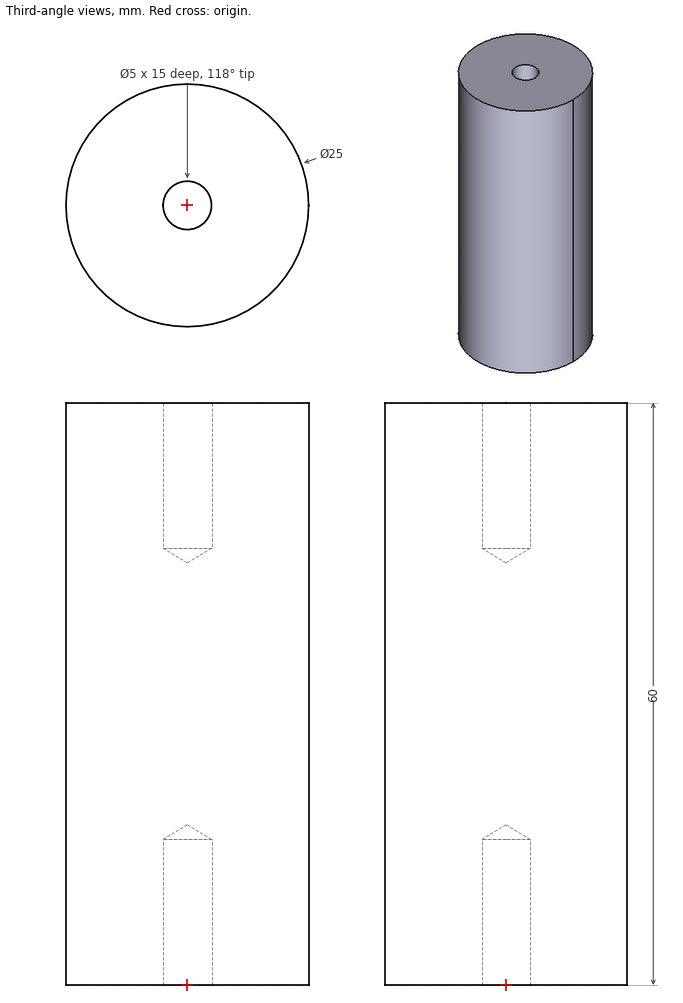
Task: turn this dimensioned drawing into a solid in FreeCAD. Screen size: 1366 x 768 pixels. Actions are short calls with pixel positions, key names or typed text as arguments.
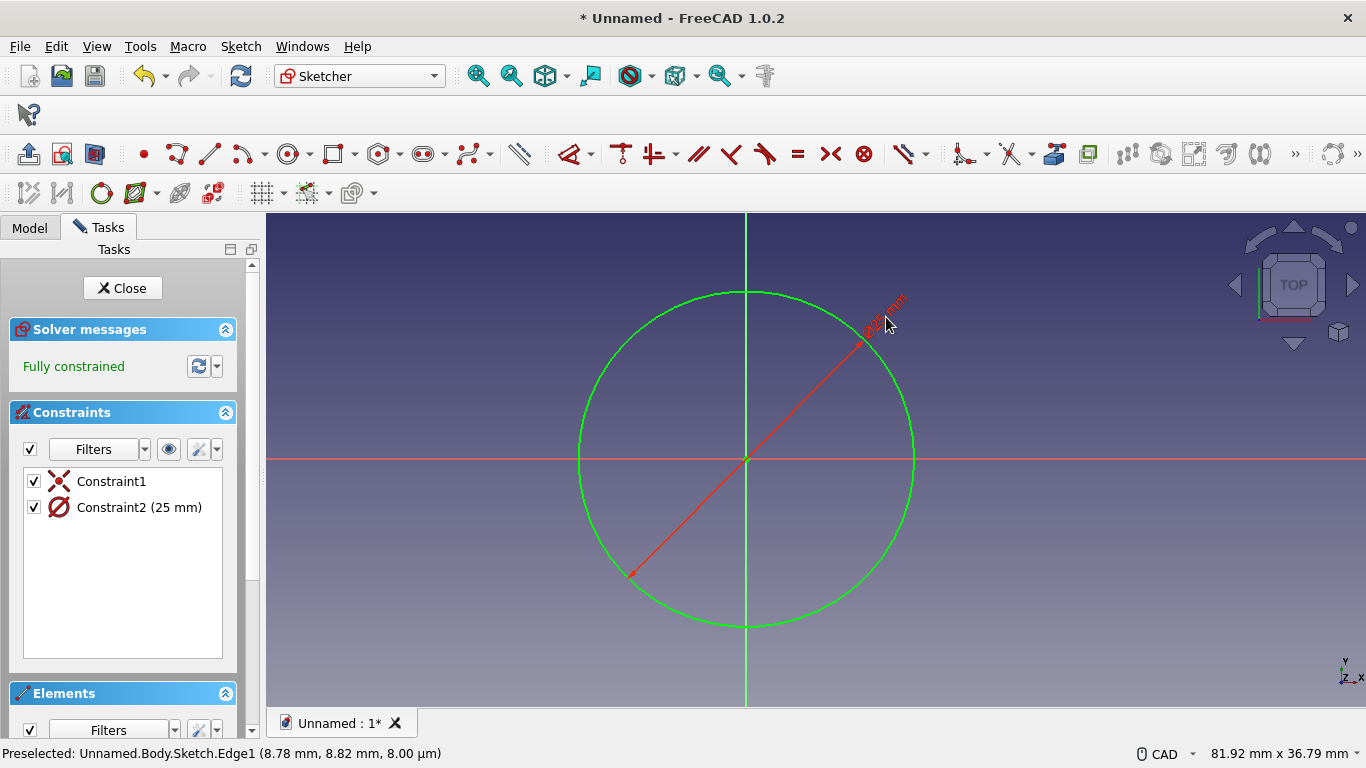
click(123, 288)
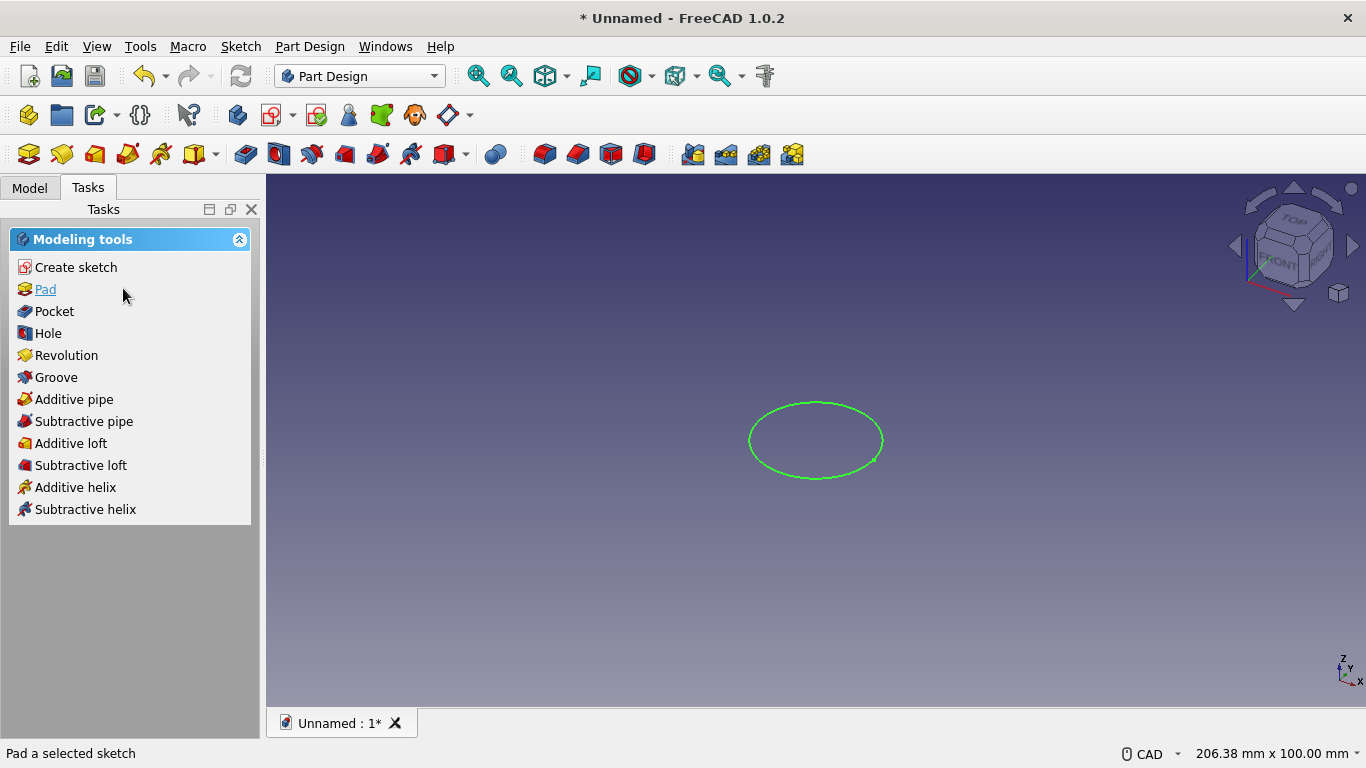
click(29, 154)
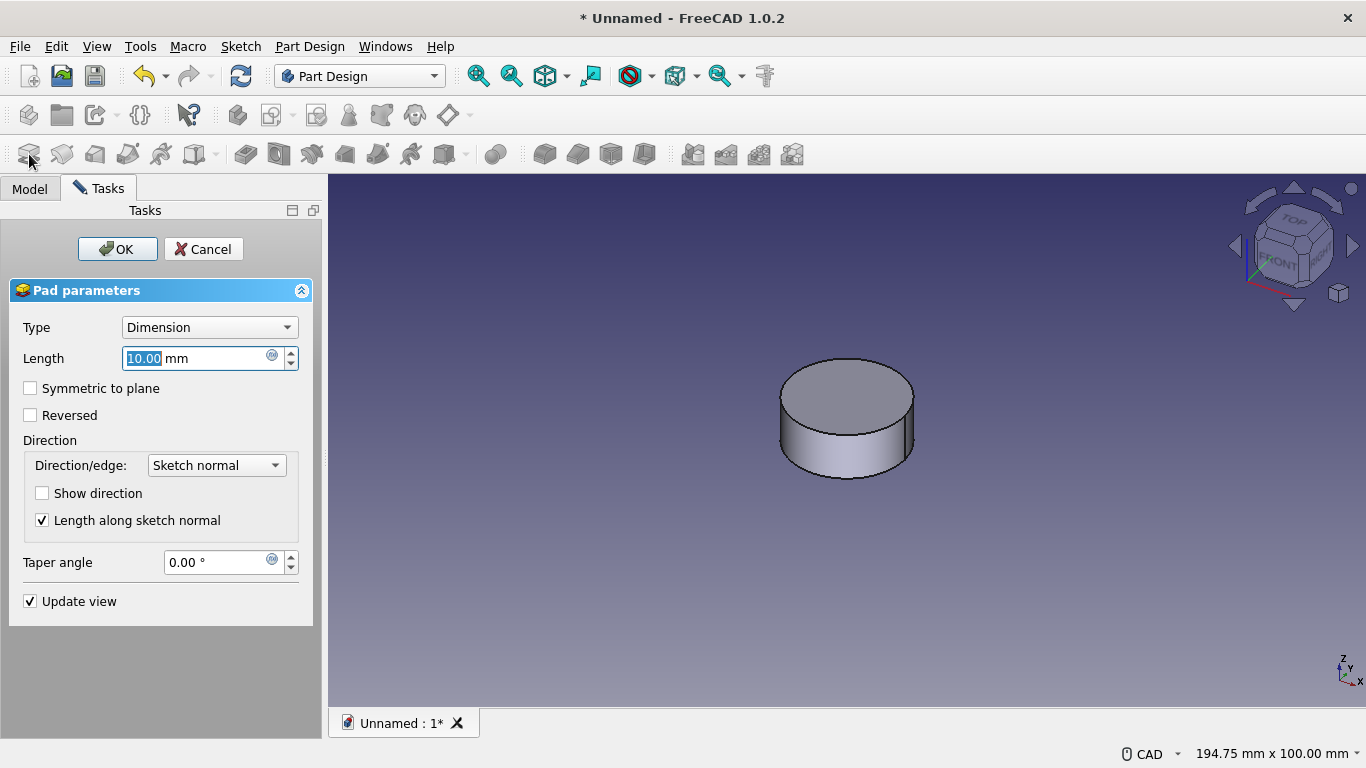
text(60)
key(Tab)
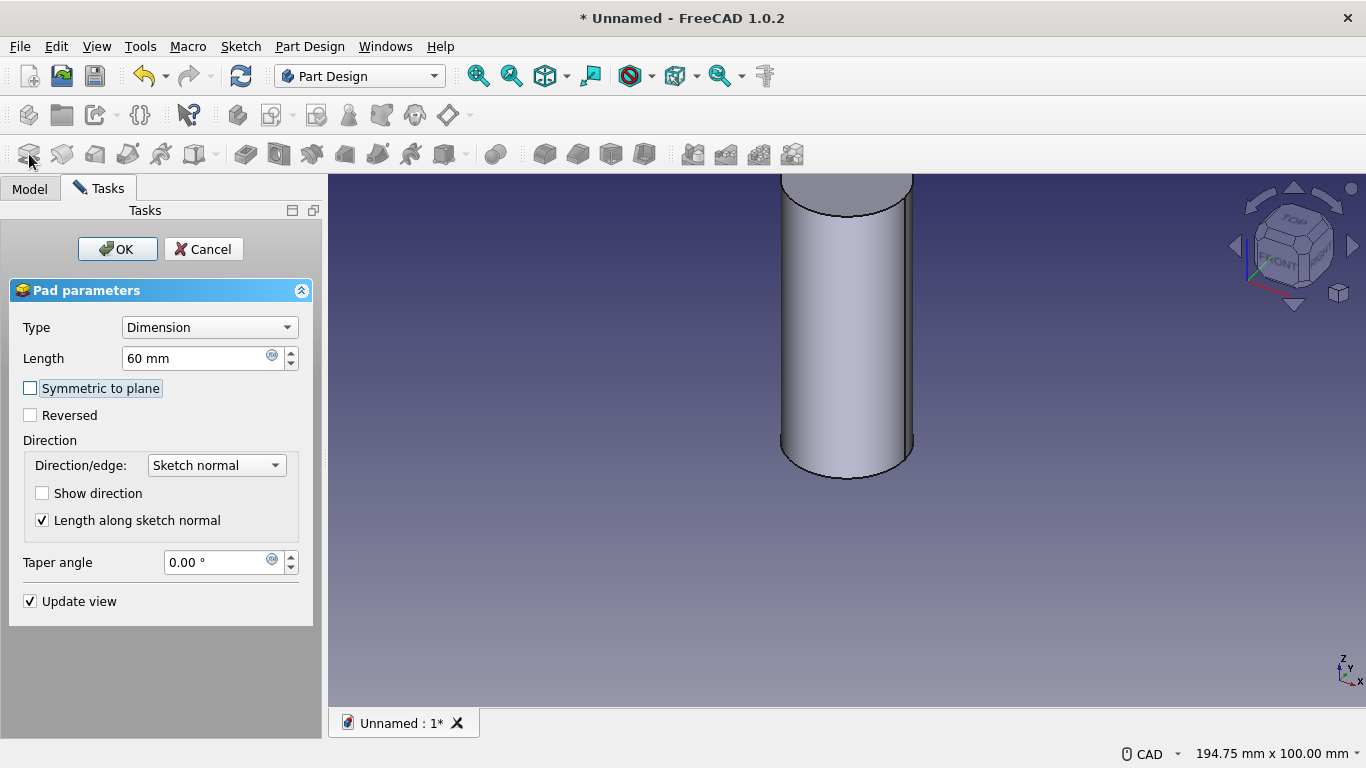
click(118, 249)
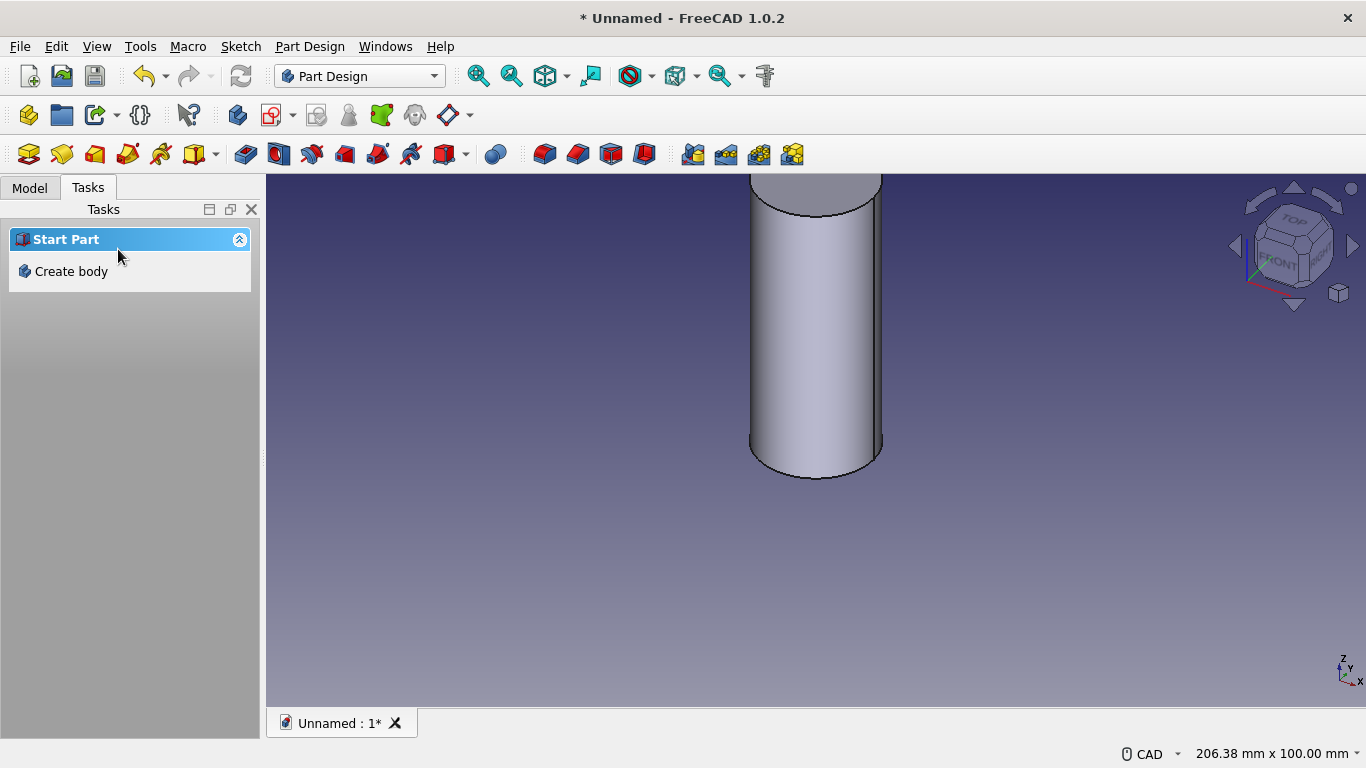
click(479, 76)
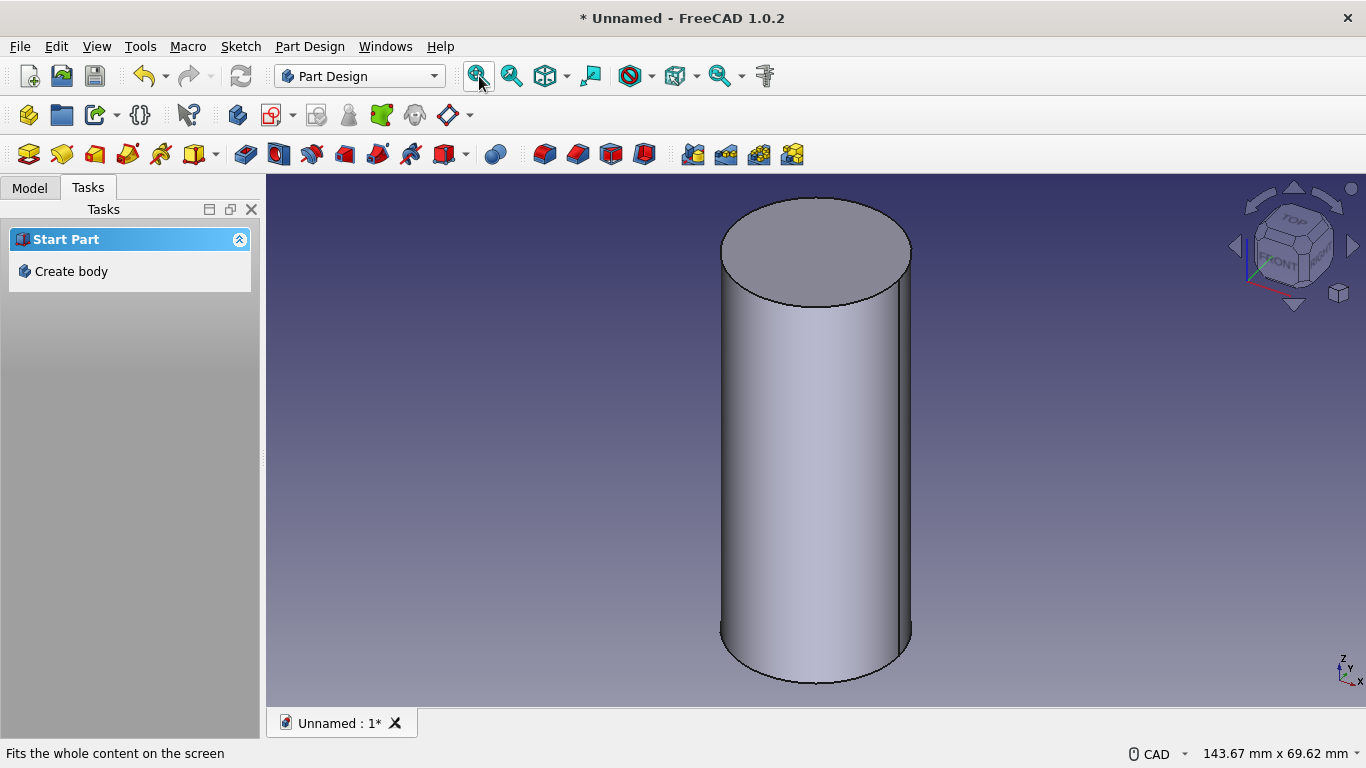
click(816, 251)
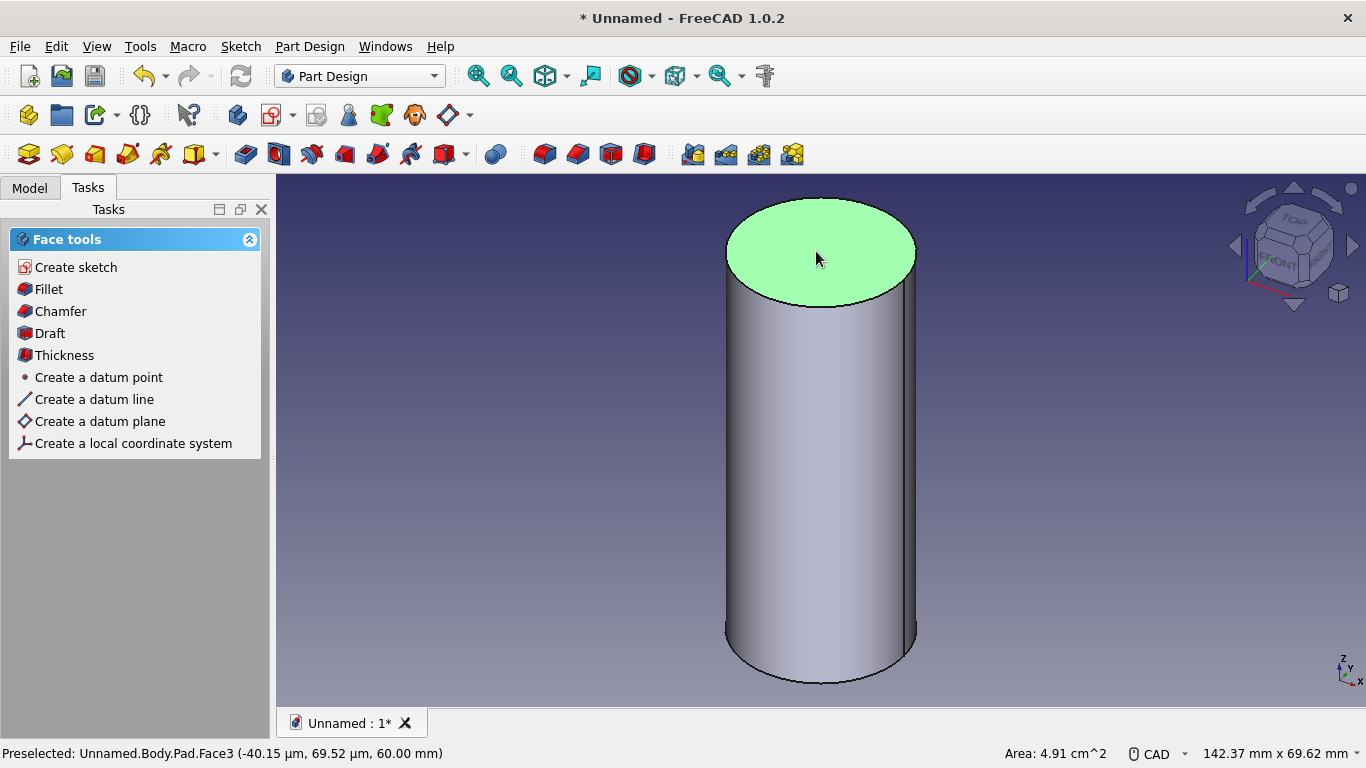
click(270, 116)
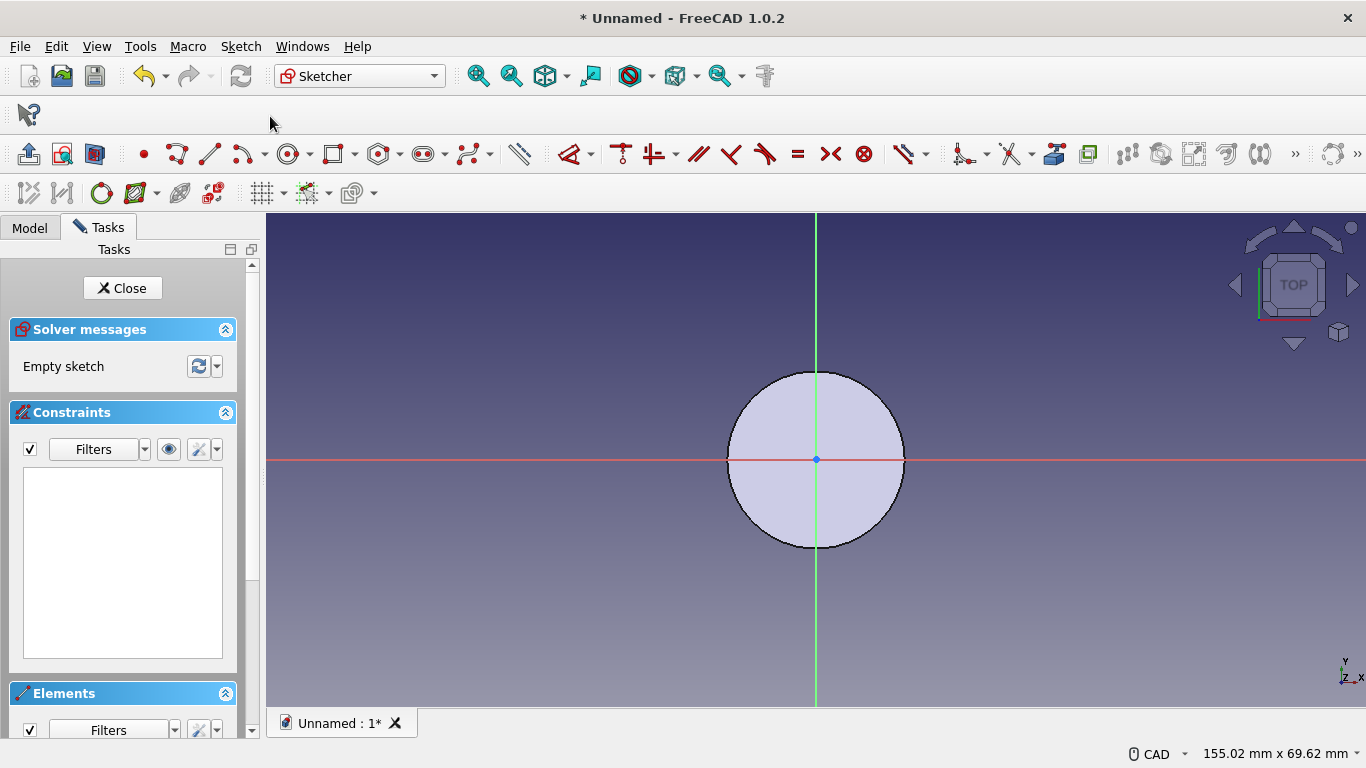
scroll(825, 460, up, 11)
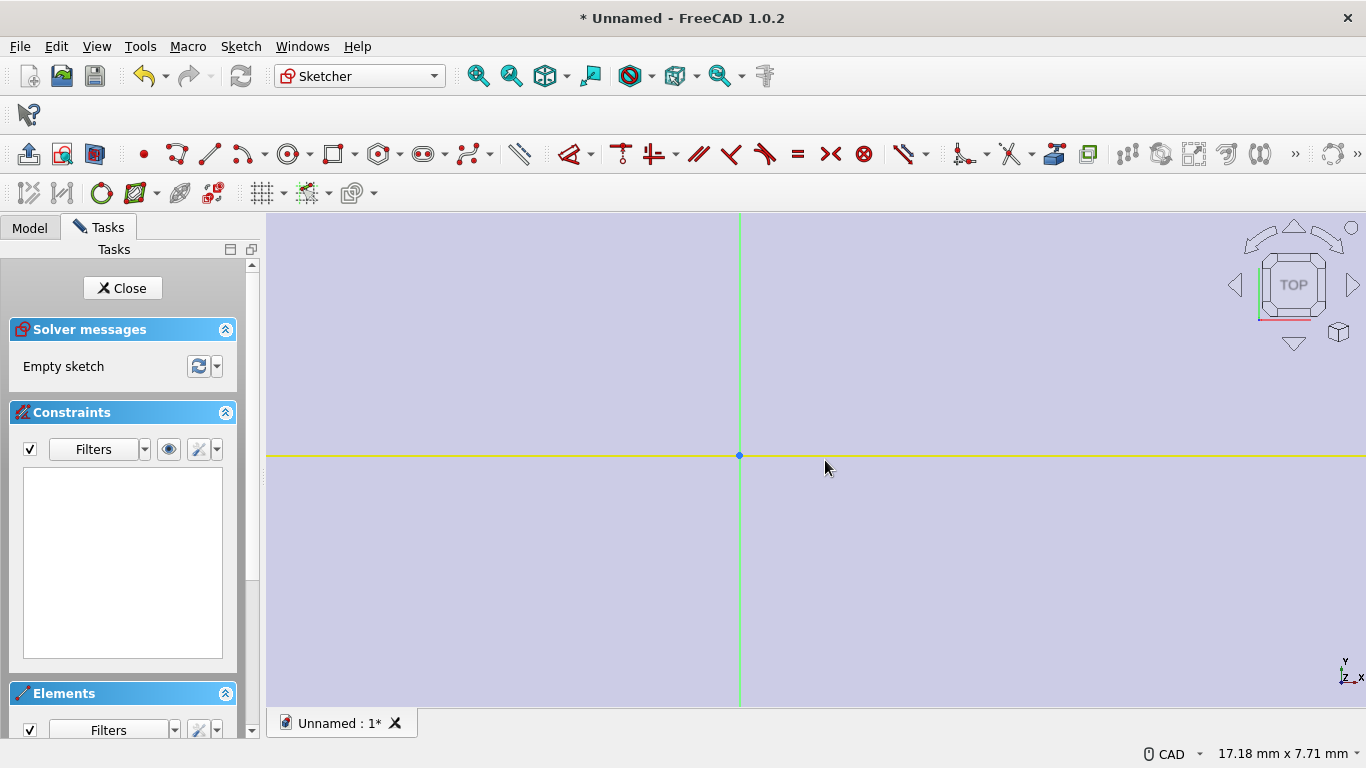
click(288, 154)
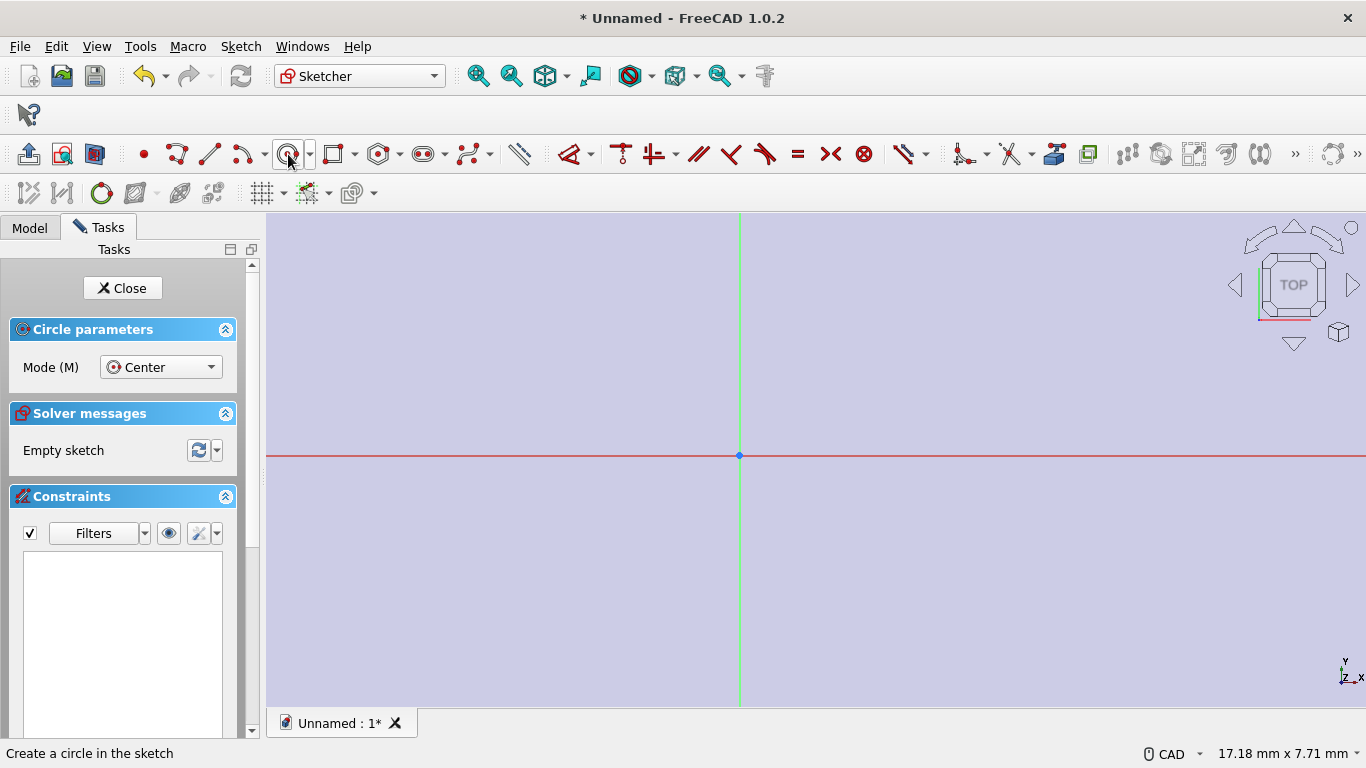
click(740, 456)
click(853, 343)
key(Escape)